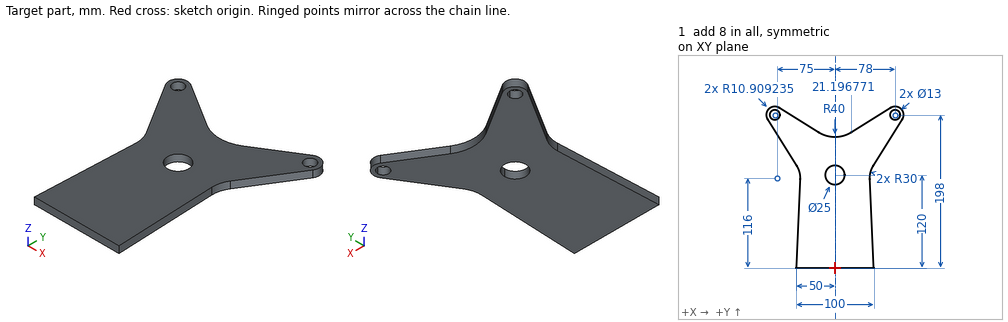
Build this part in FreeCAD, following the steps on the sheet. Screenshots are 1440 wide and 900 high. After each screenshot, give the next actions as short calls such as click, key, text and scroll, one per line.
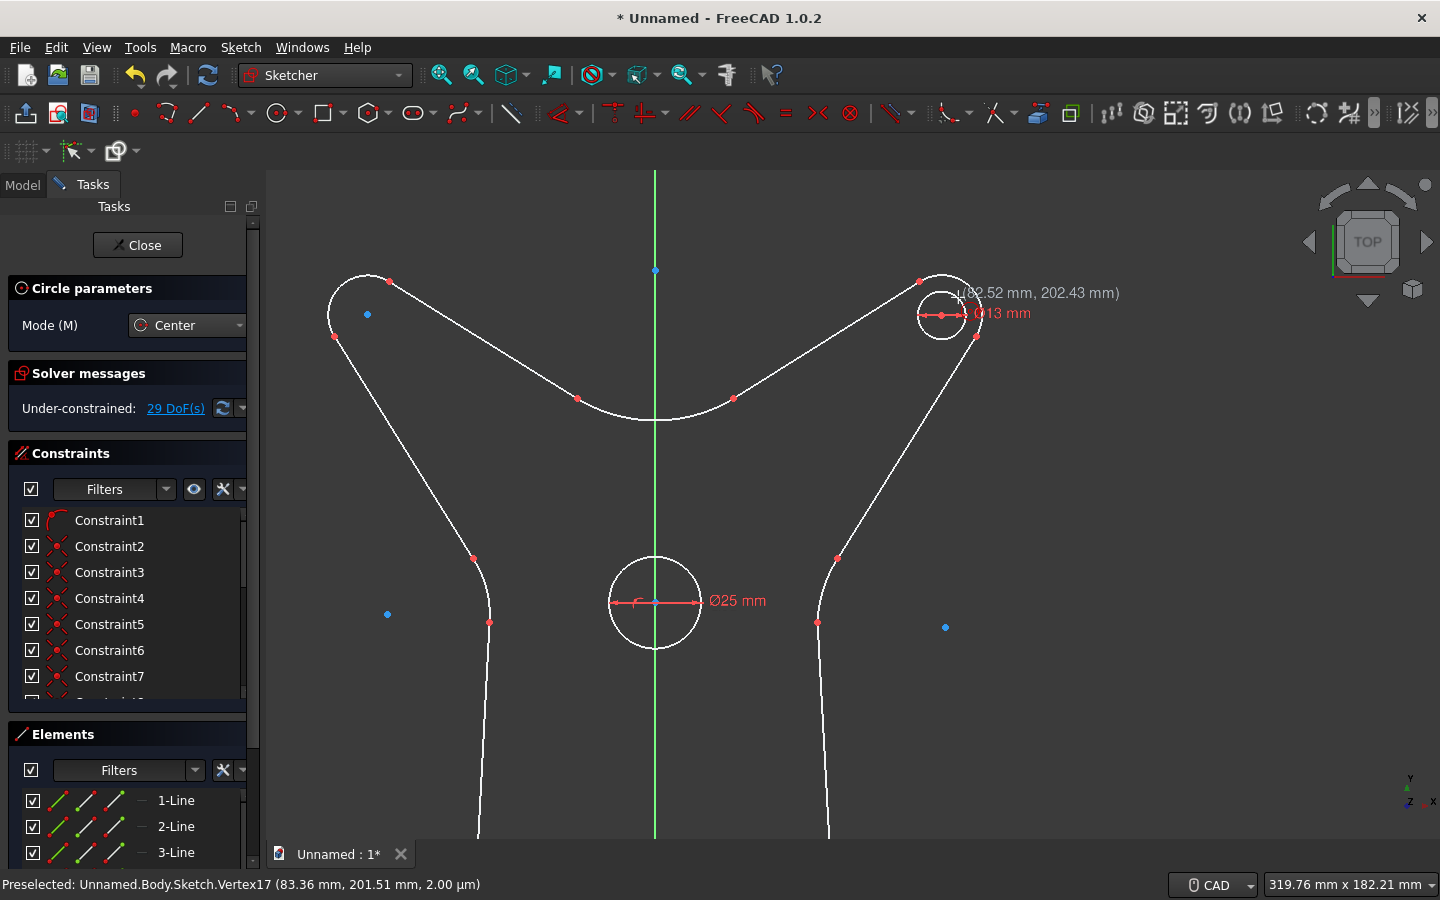
click(369, 314)
move(386, 297)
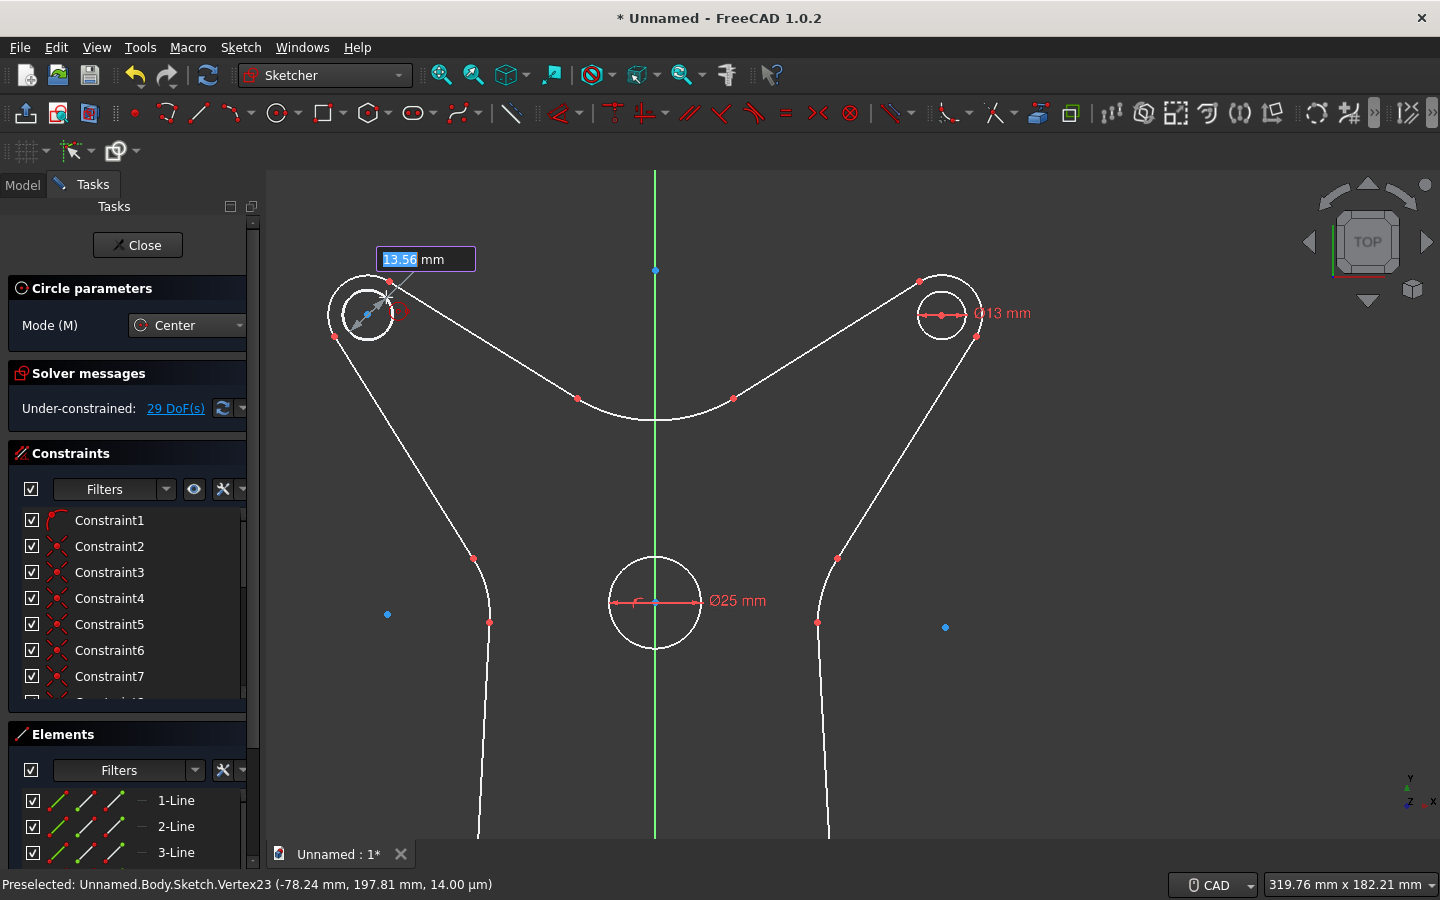
text(13)
key(Return)
key(Escape)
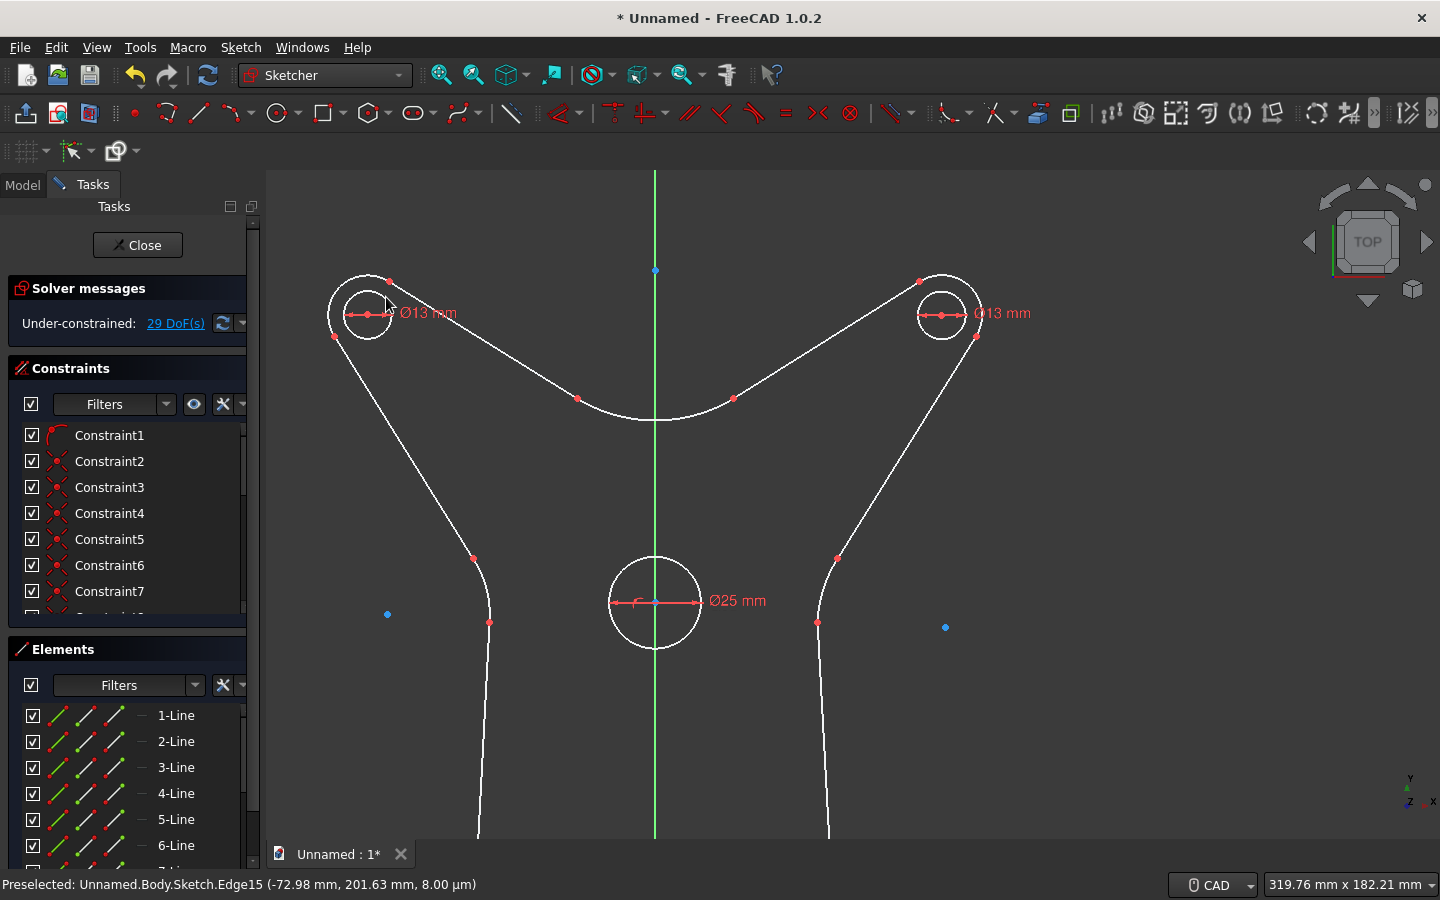
click(879, 492)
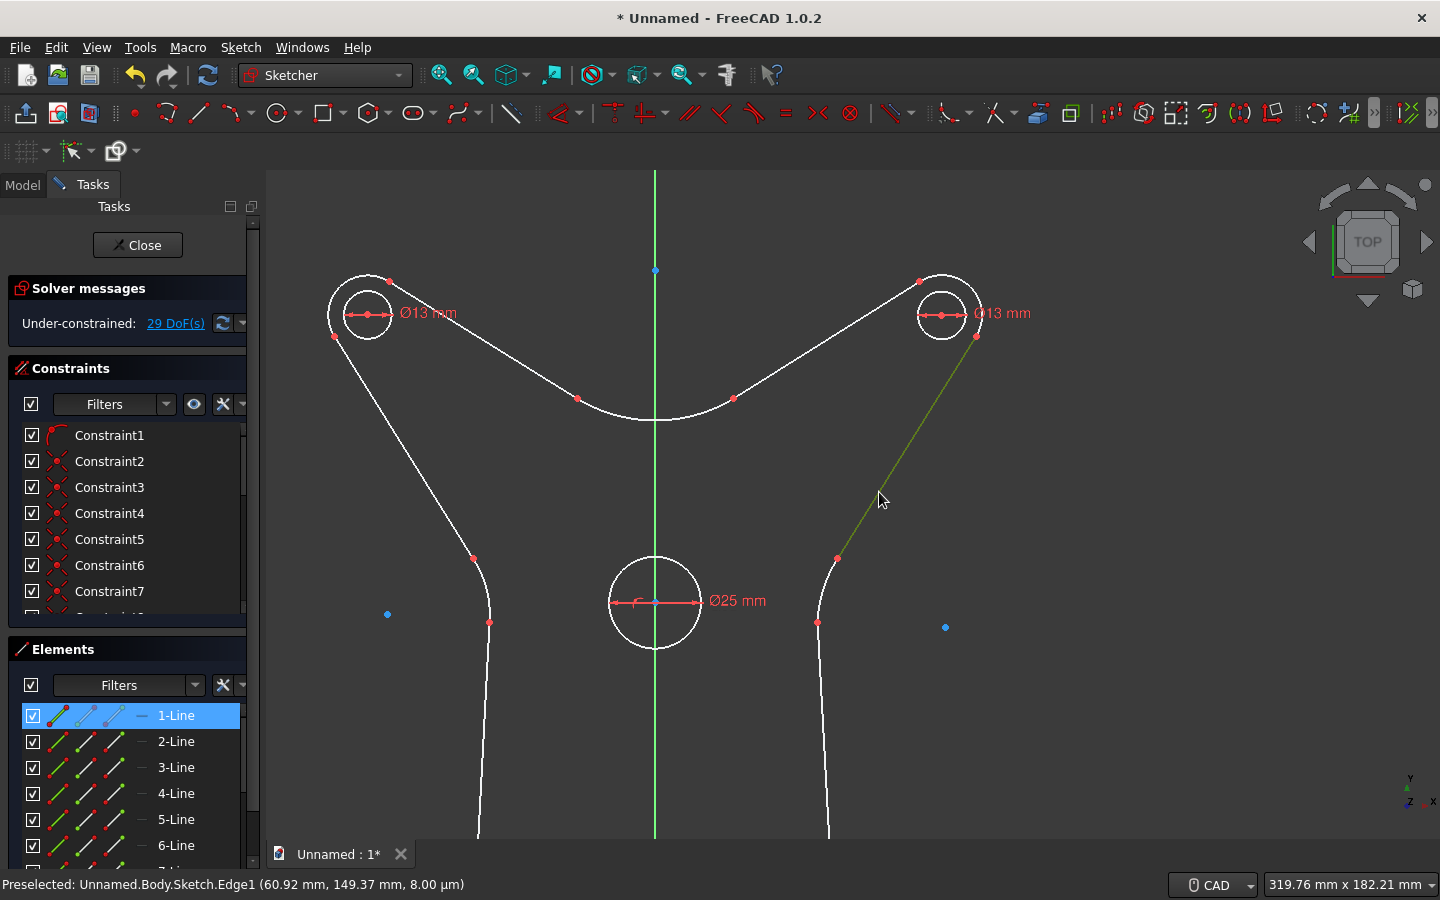
click(981, 305)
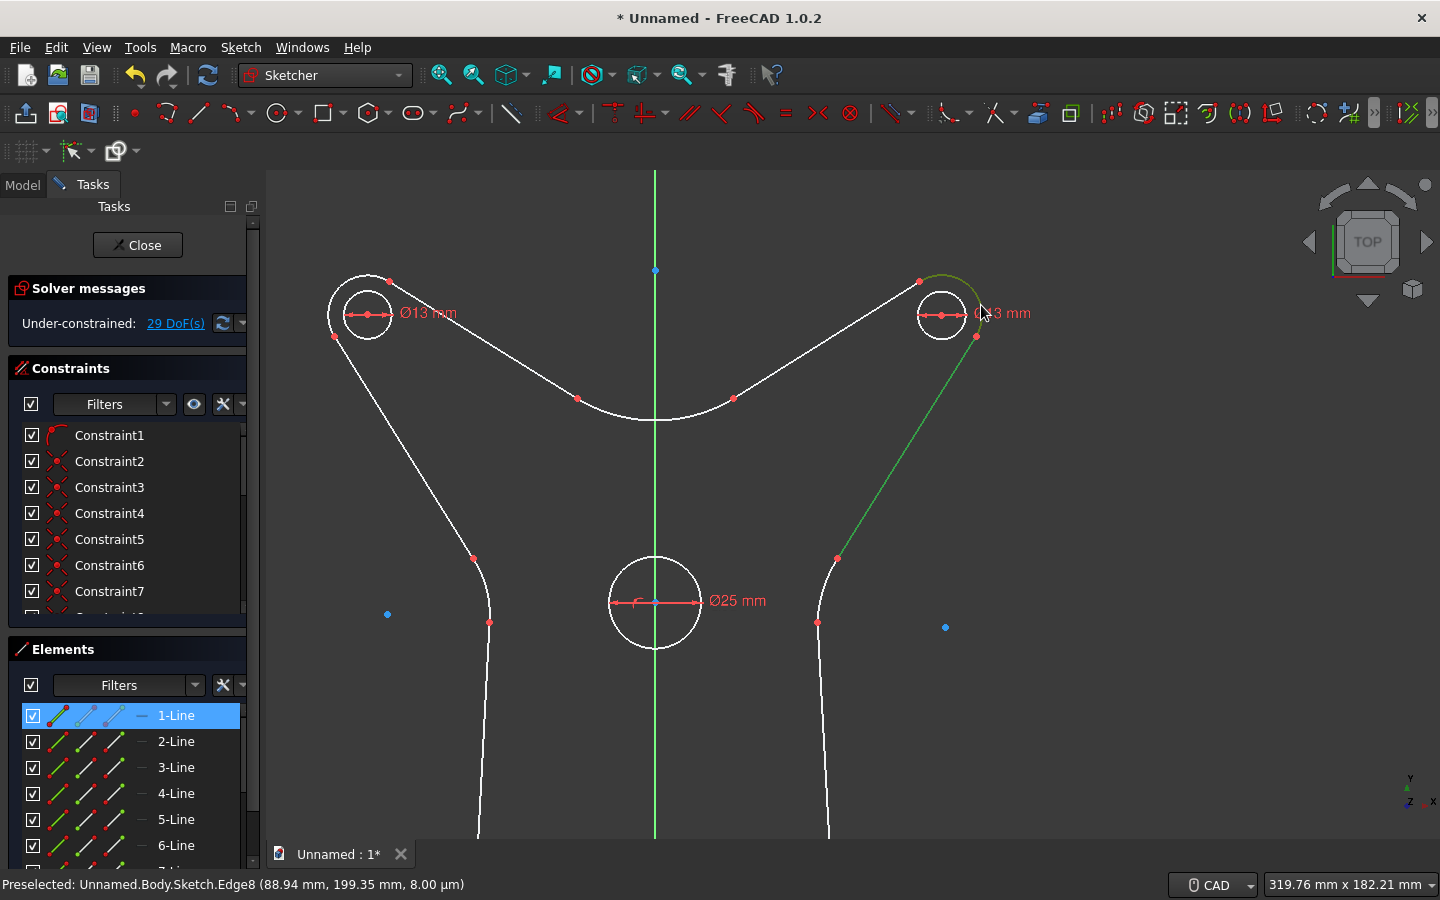
click(754, 114)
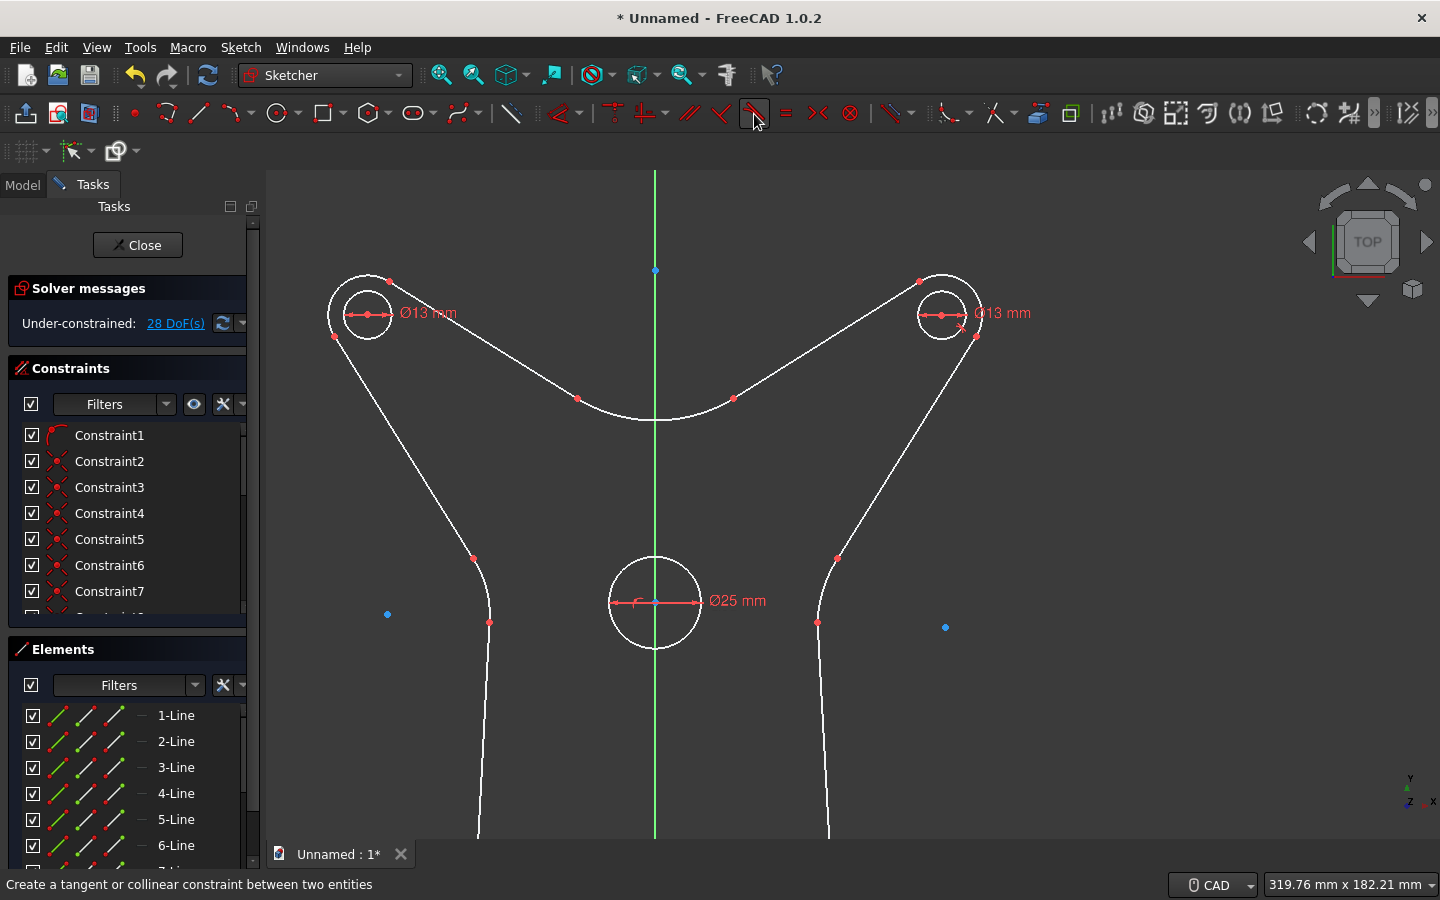
click(879, 492)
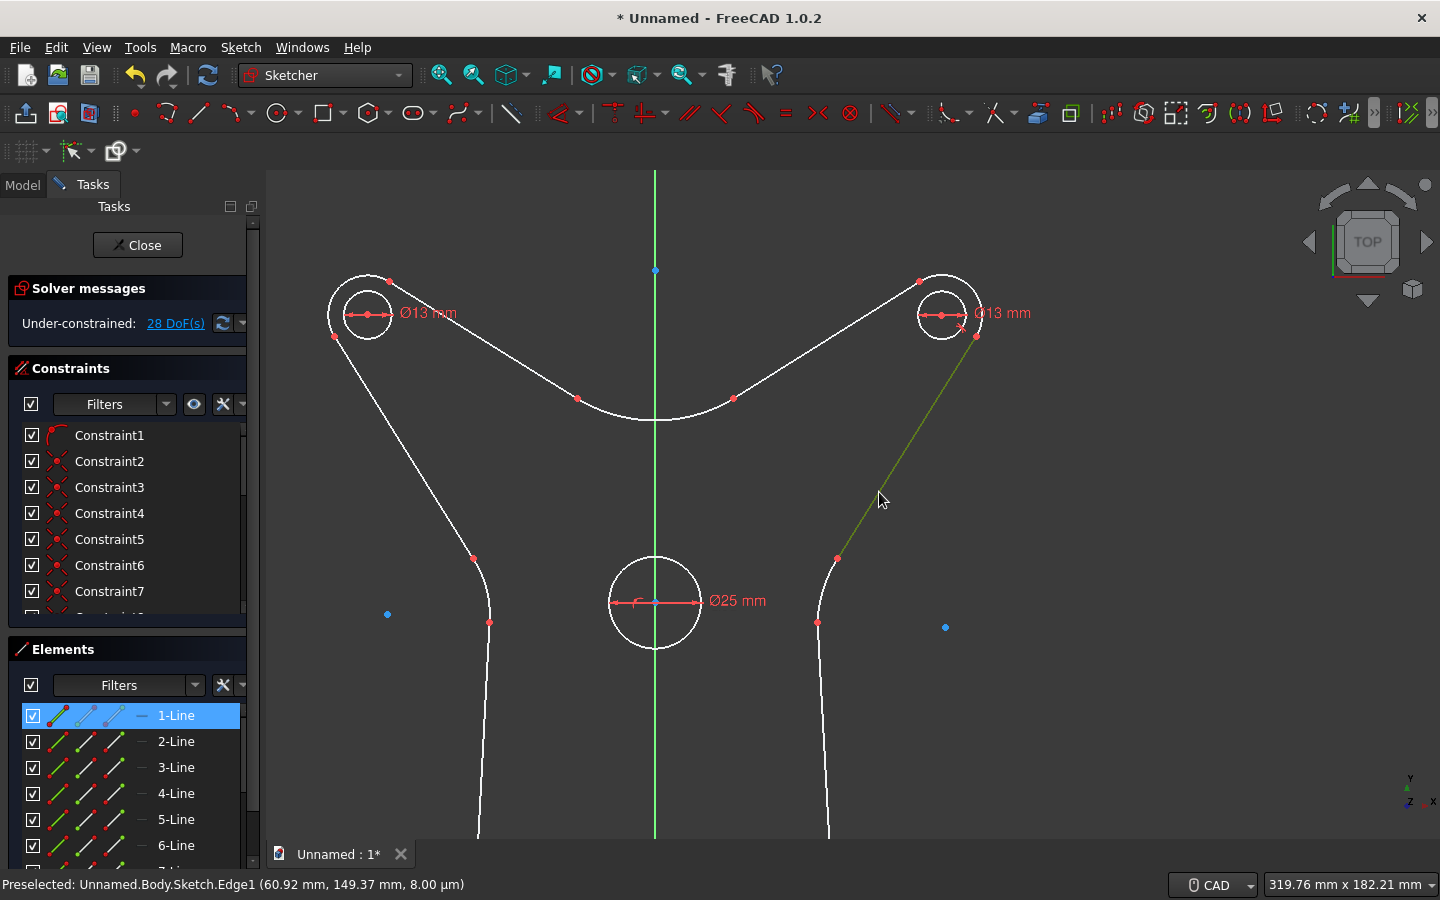
click(828, 577)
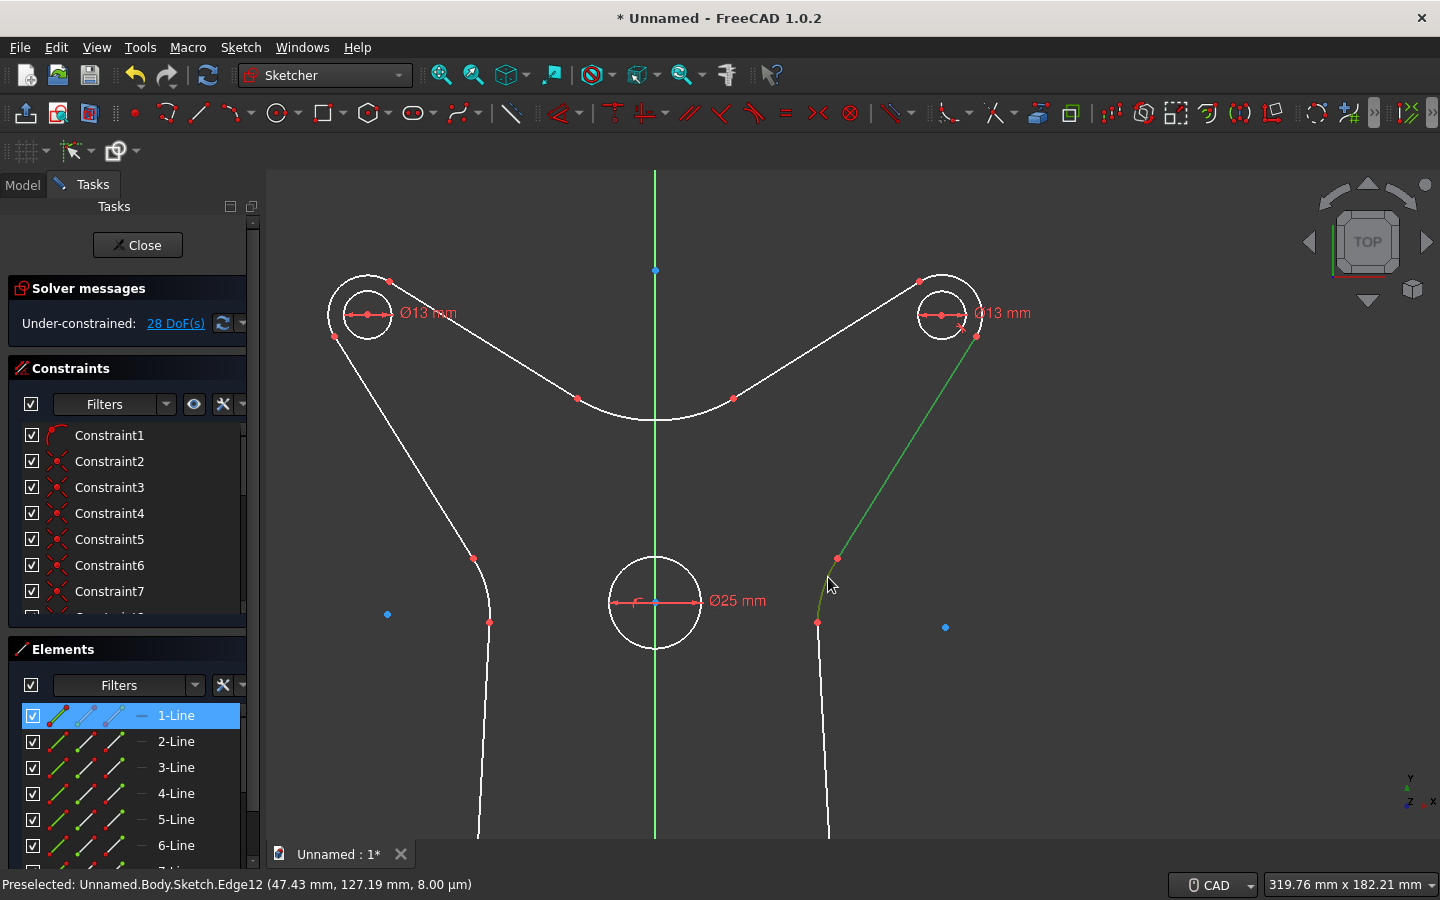
click(754, 114)